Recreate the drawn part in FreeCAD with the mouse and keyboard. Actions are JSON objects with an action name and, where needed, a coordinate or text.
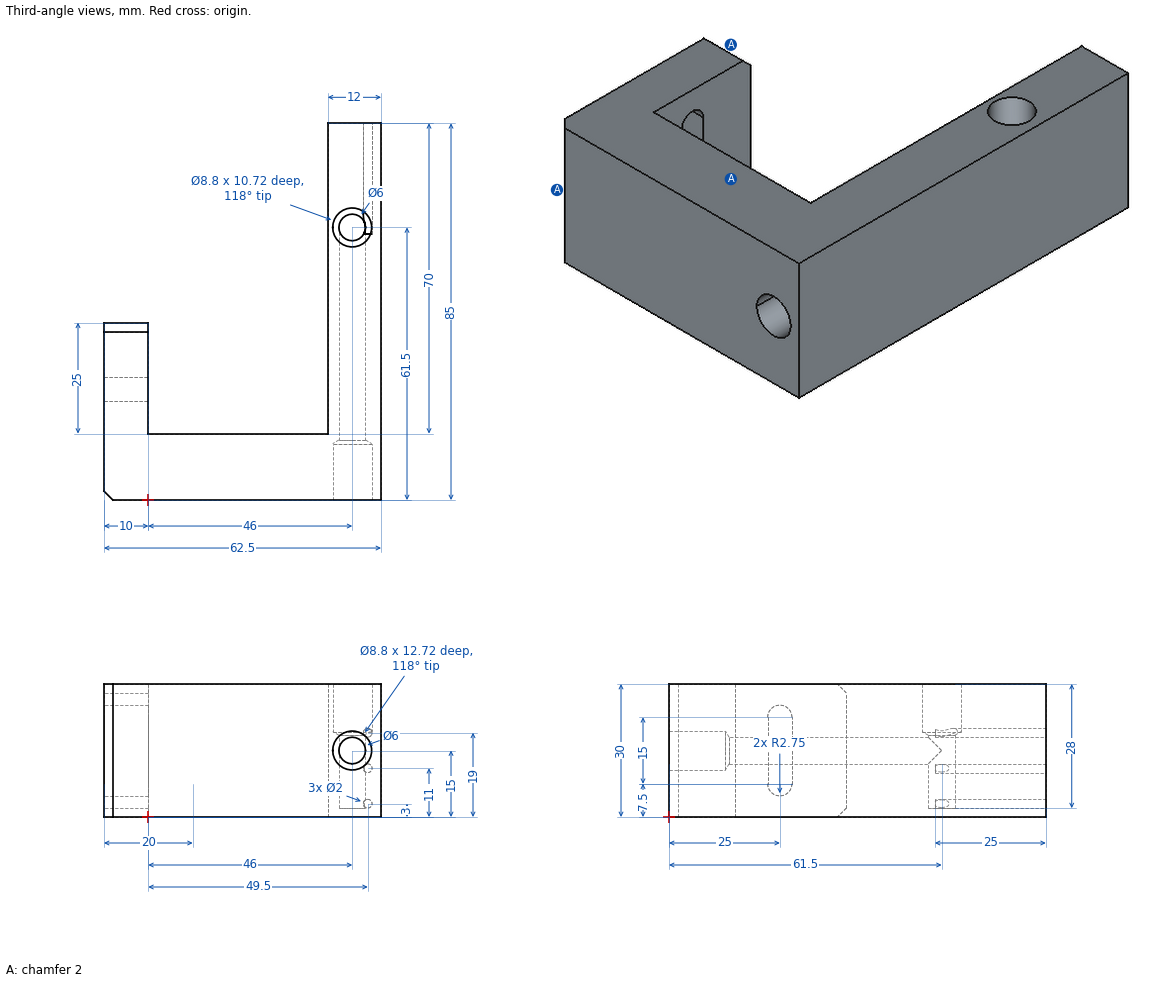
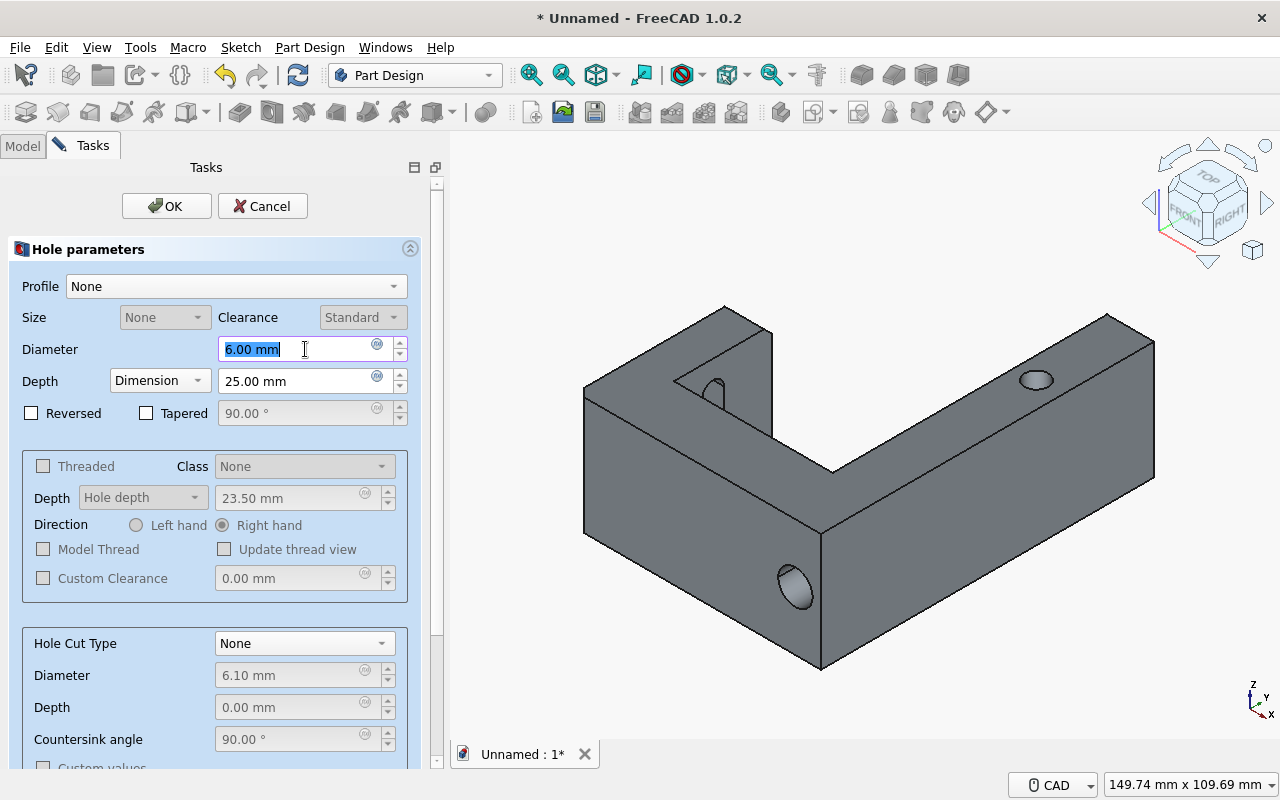
{"action": "type", "text": "8.8"}
{"action": "key", "text": "Tab"}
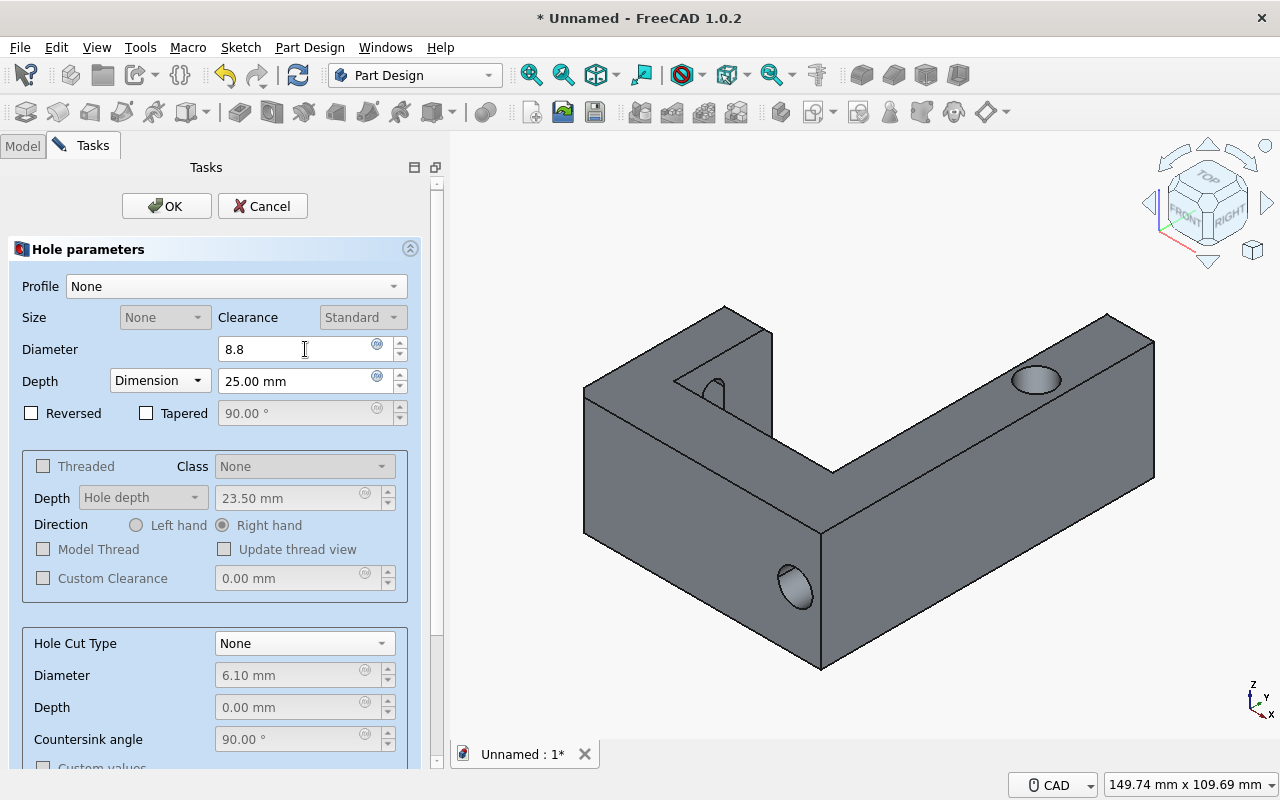
{"action": "triple_click", "coordinate": [305, 381]}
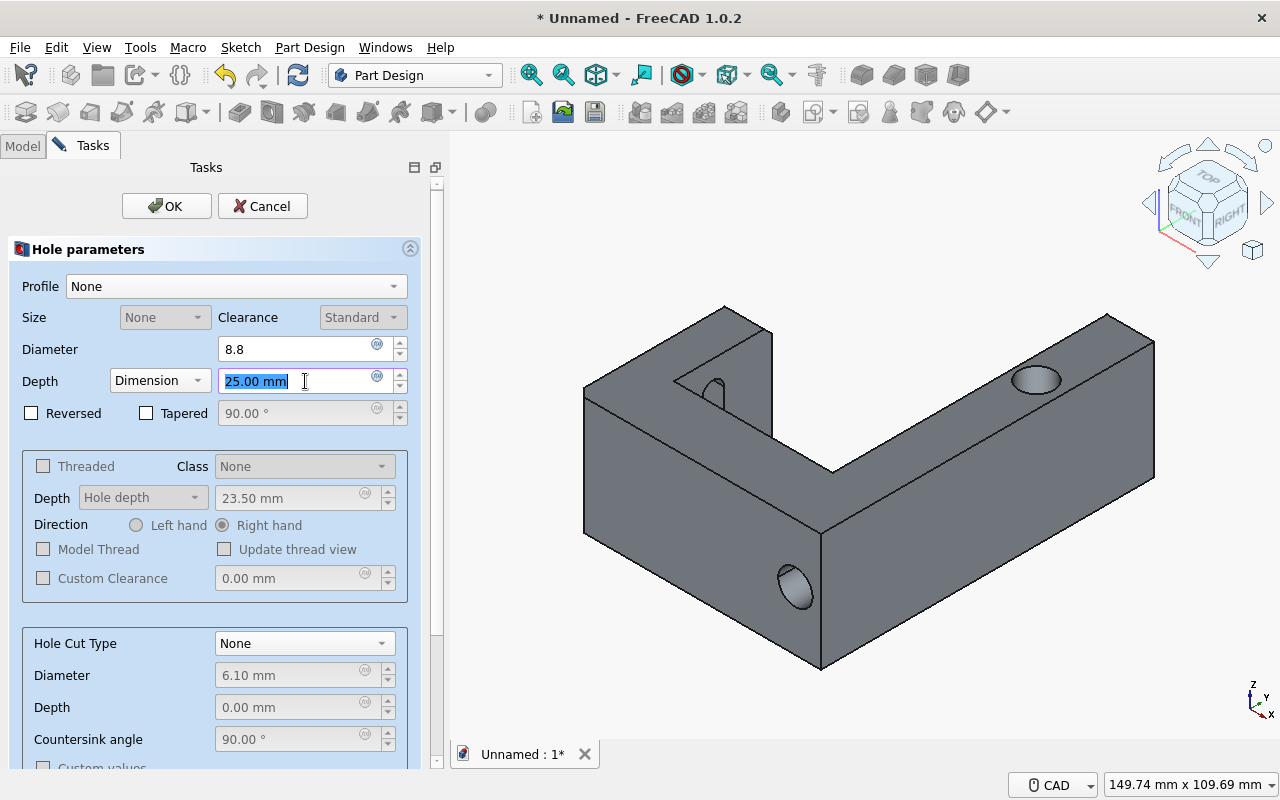
{"action": "type", "text": "10.72"}
{"action": "key", "text": "Tab"}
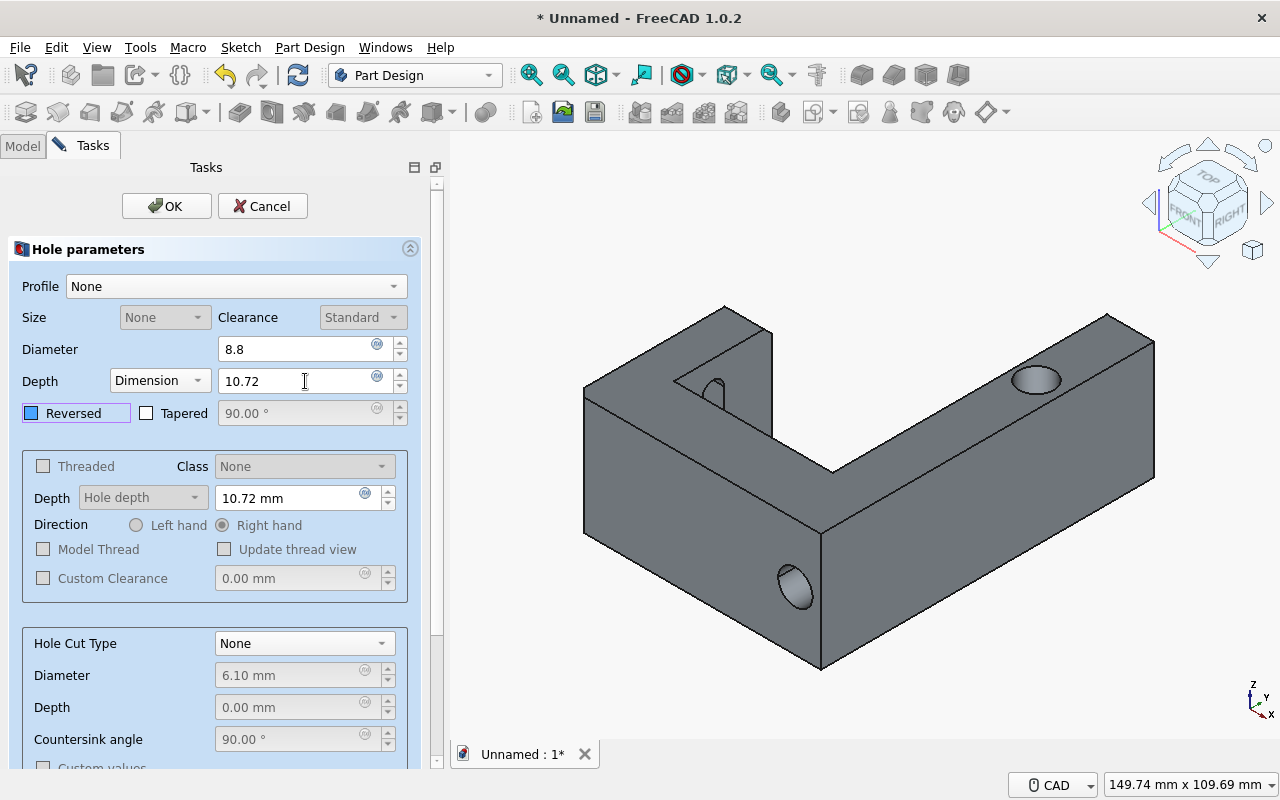
{"action": "left_click", "coordinate": [167, 206]}